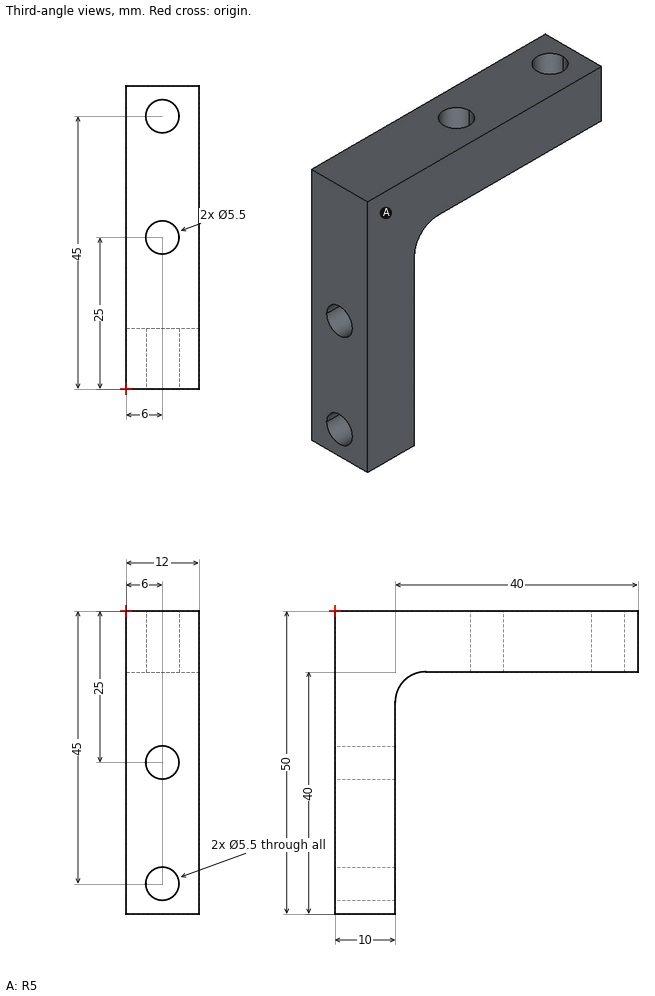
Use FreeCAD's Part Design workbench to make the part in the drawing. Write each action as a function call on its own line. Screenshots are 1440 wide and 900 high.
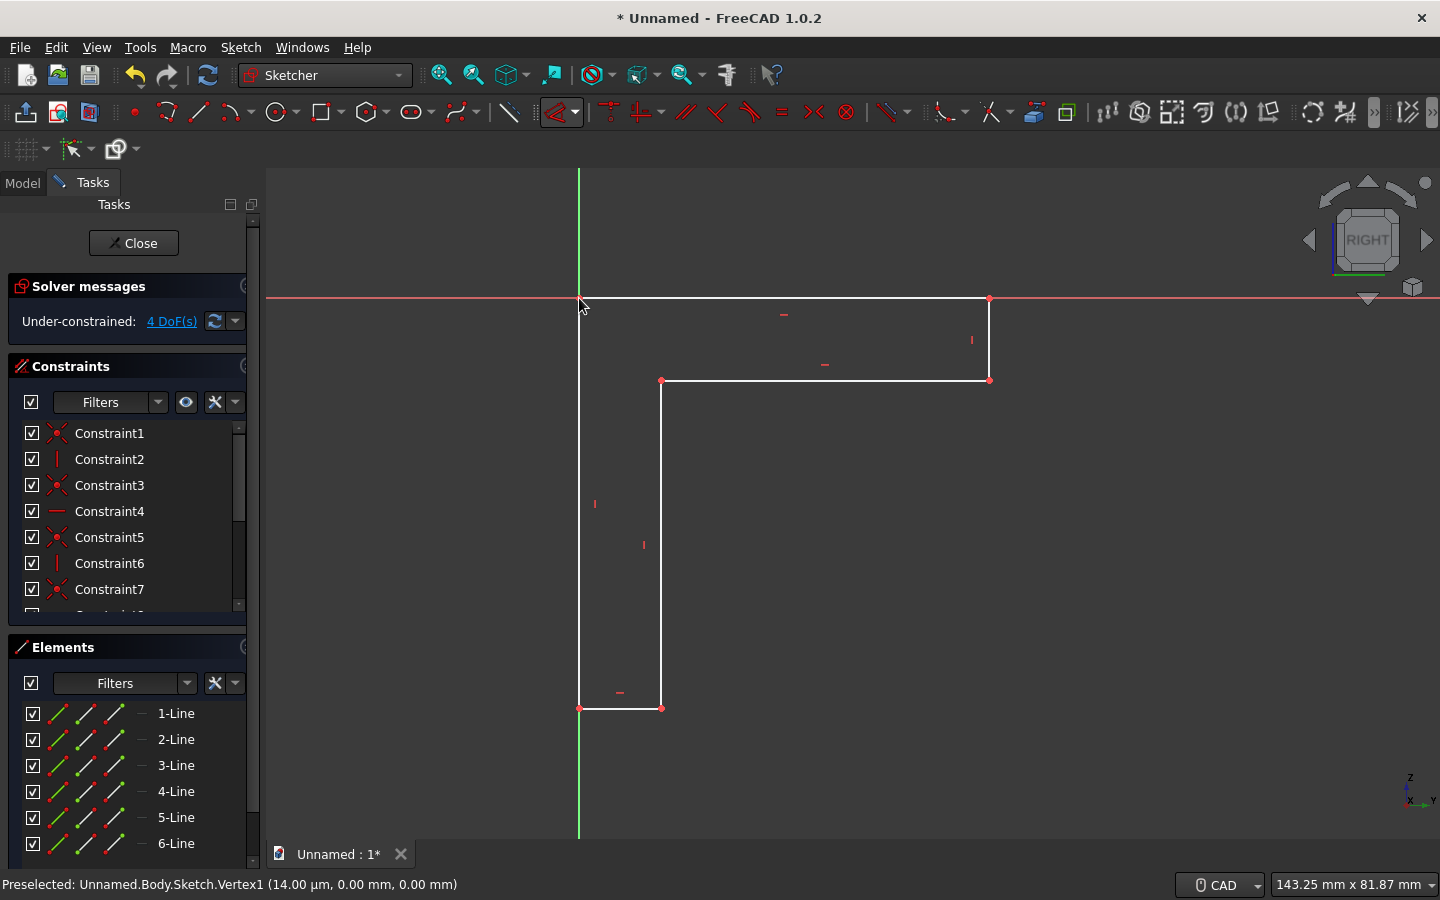
click(556, 112)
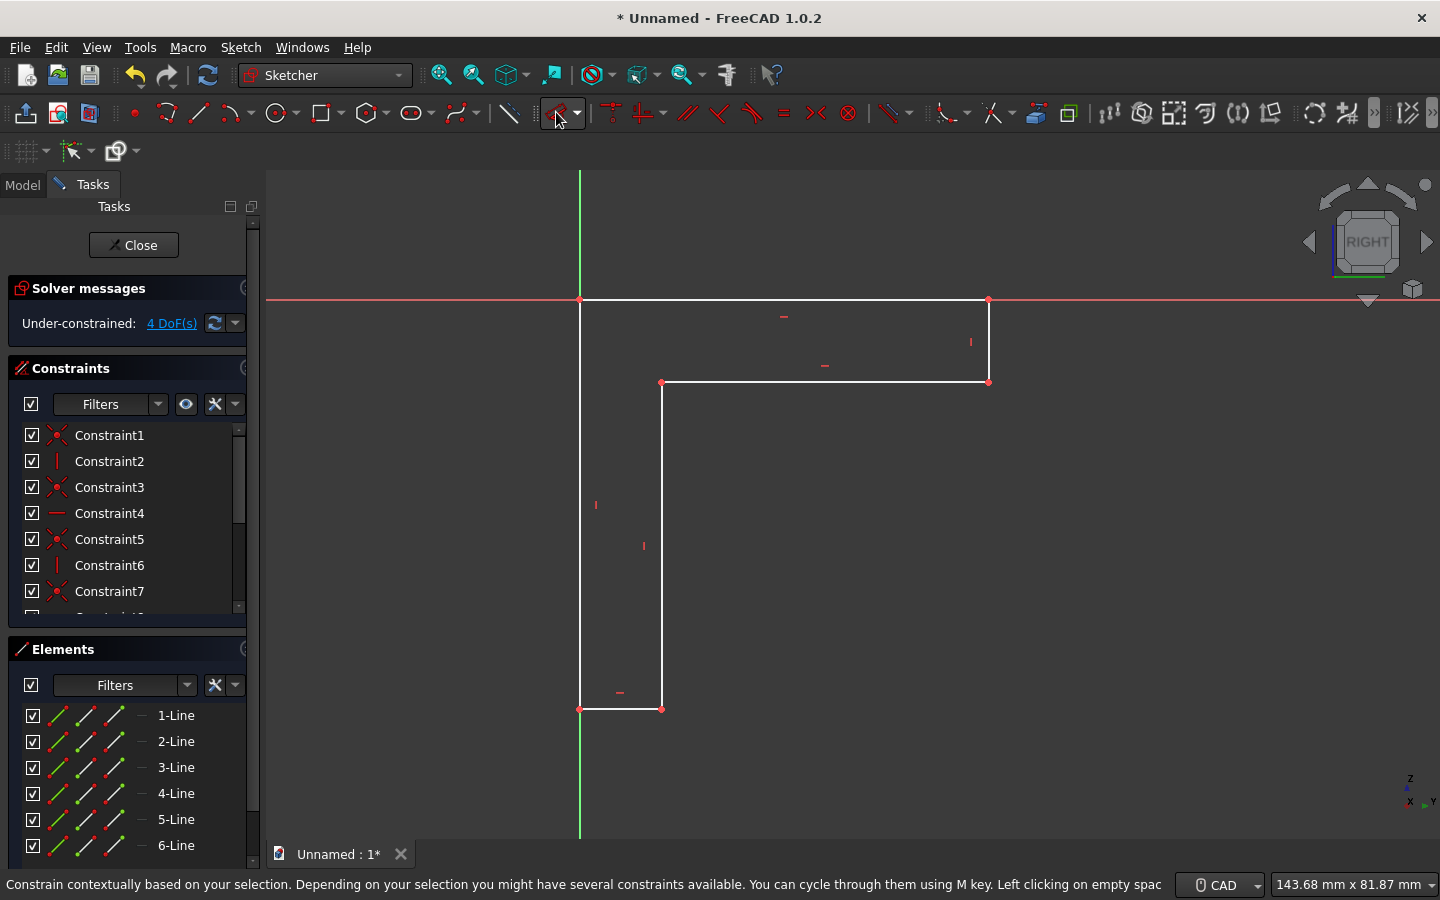
click(580, 423)
click(546, 505)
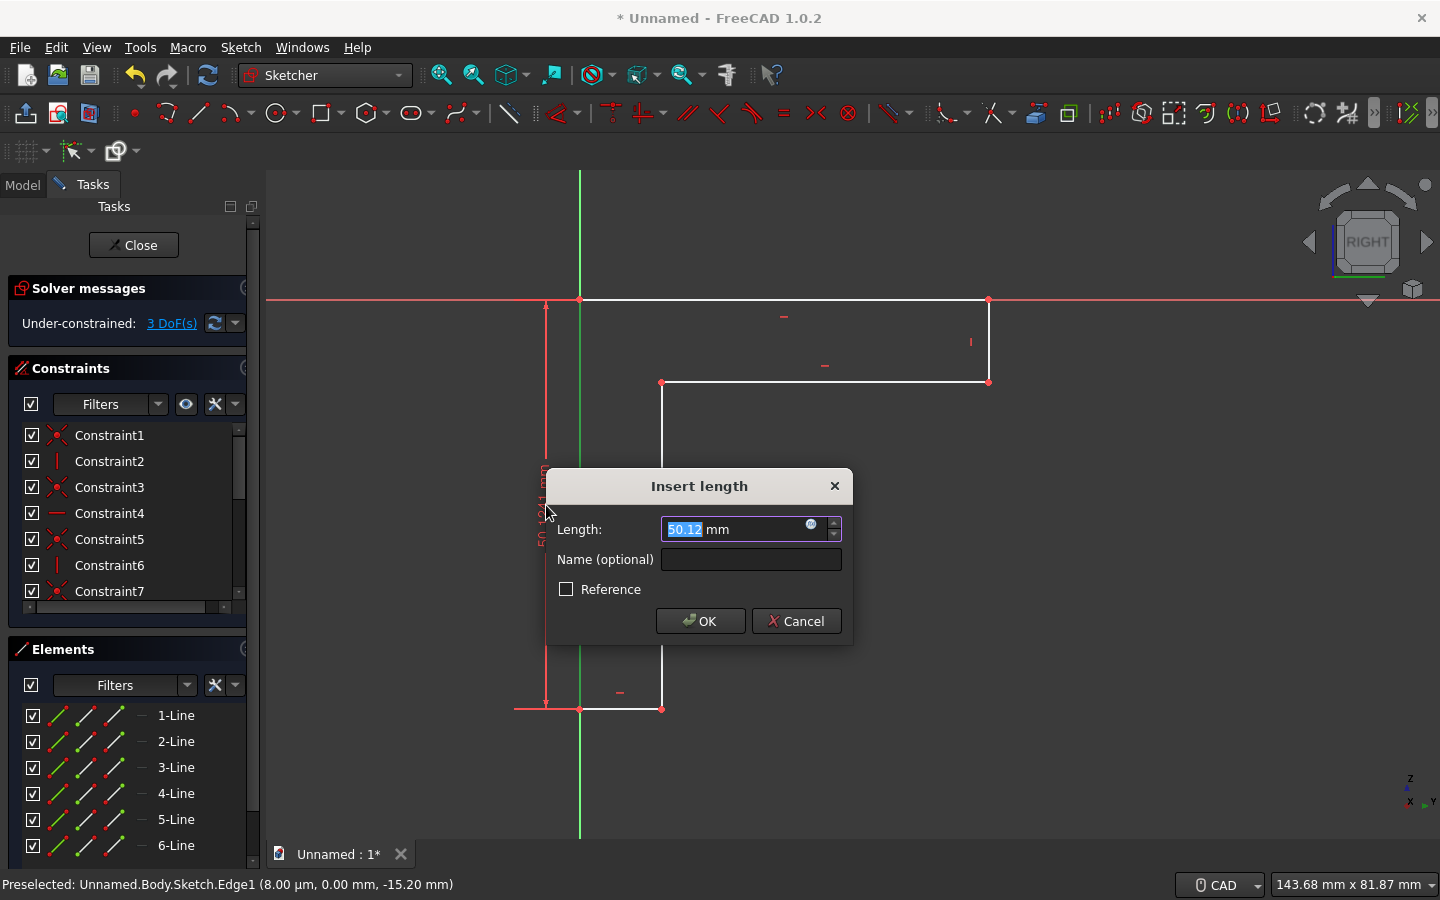
text(50)
key(Return)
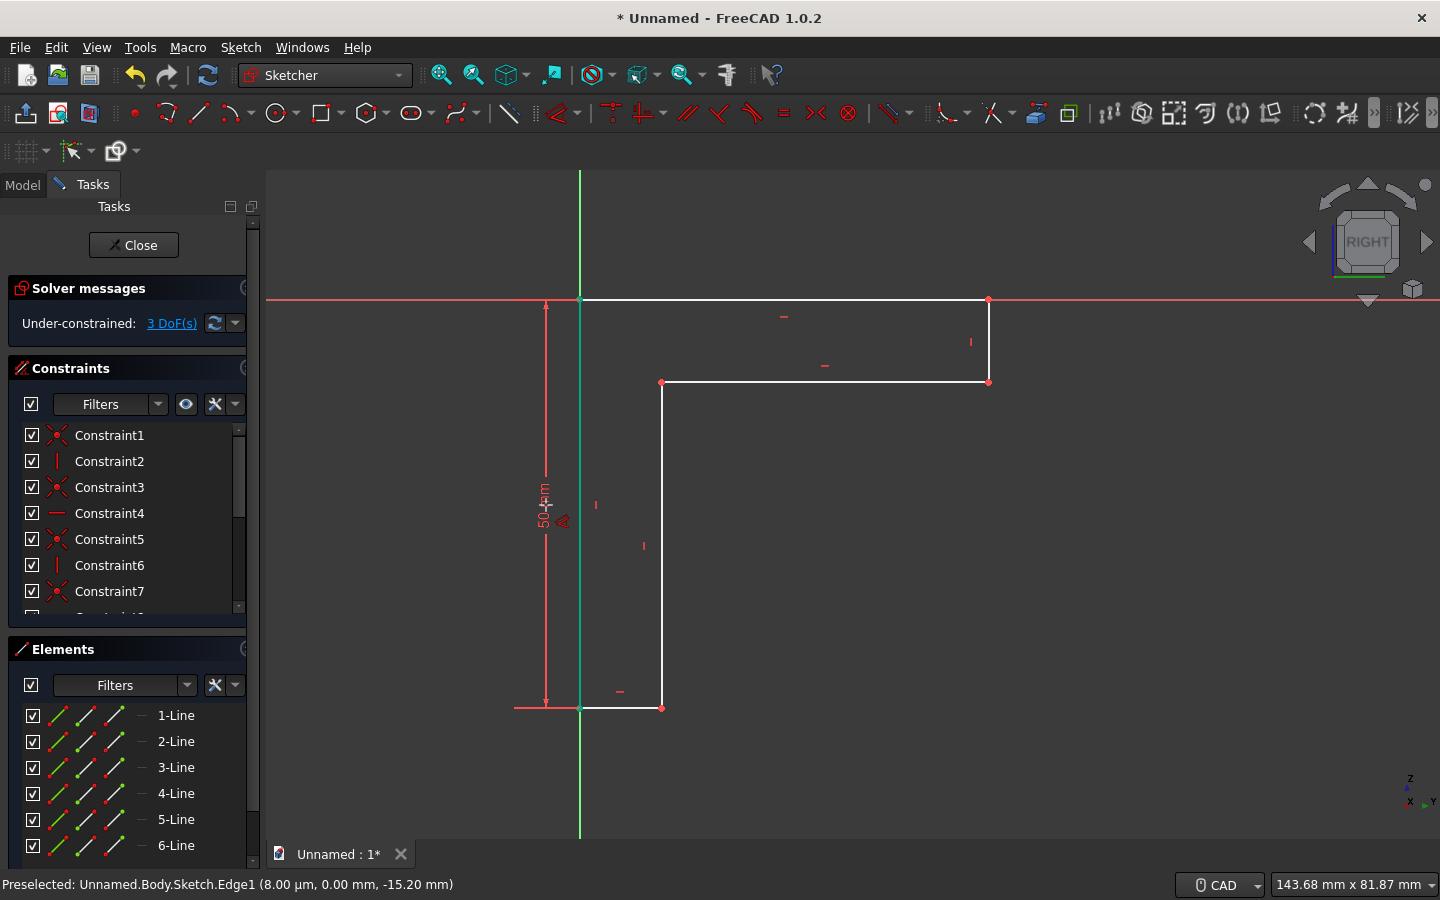
click(604, 708)
click(621, 742)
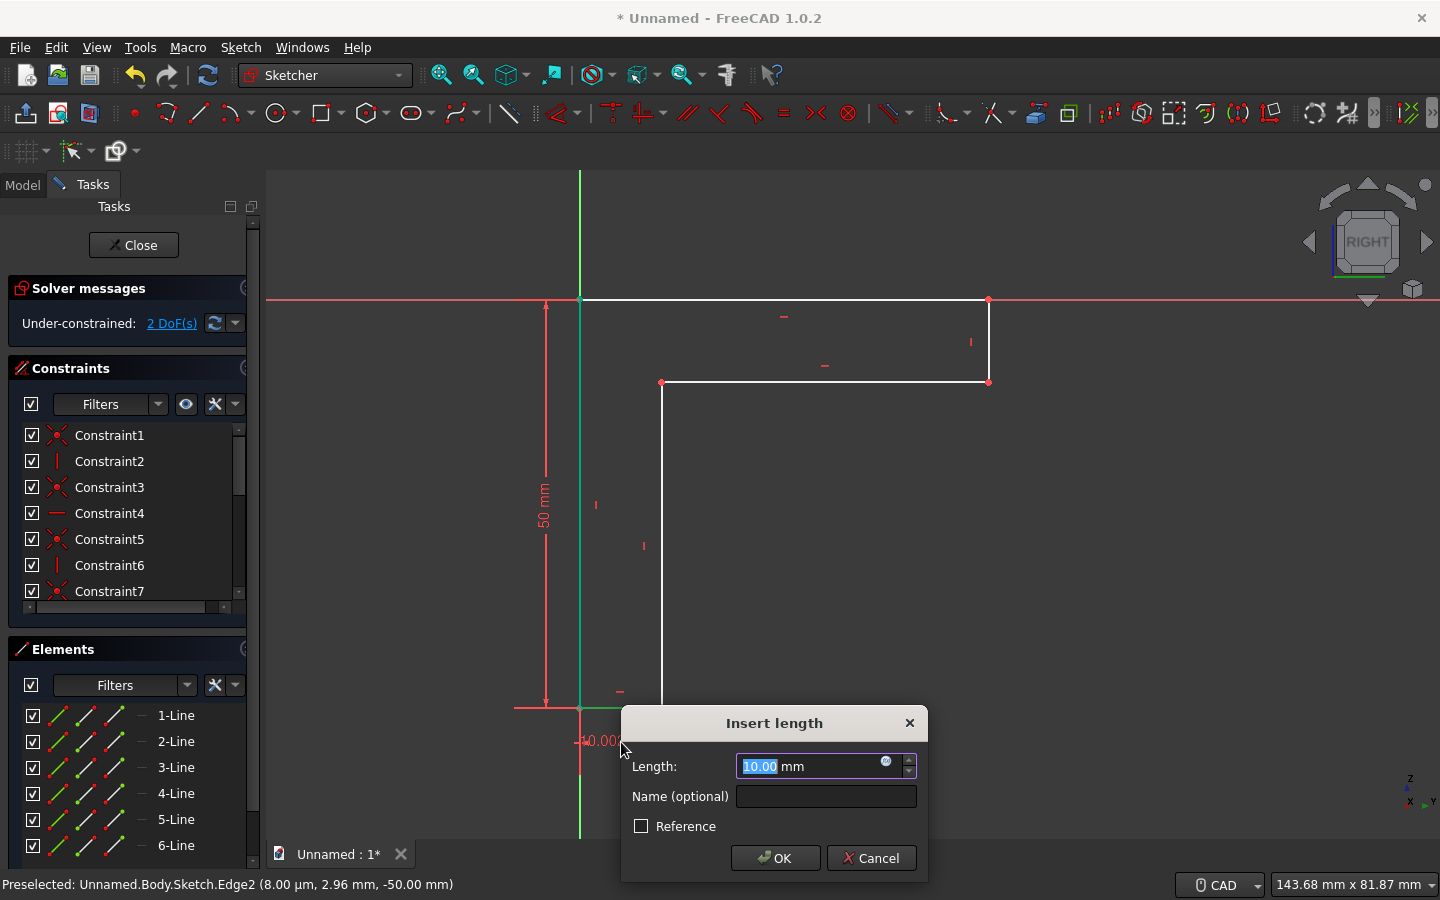
text(10)
key(Return)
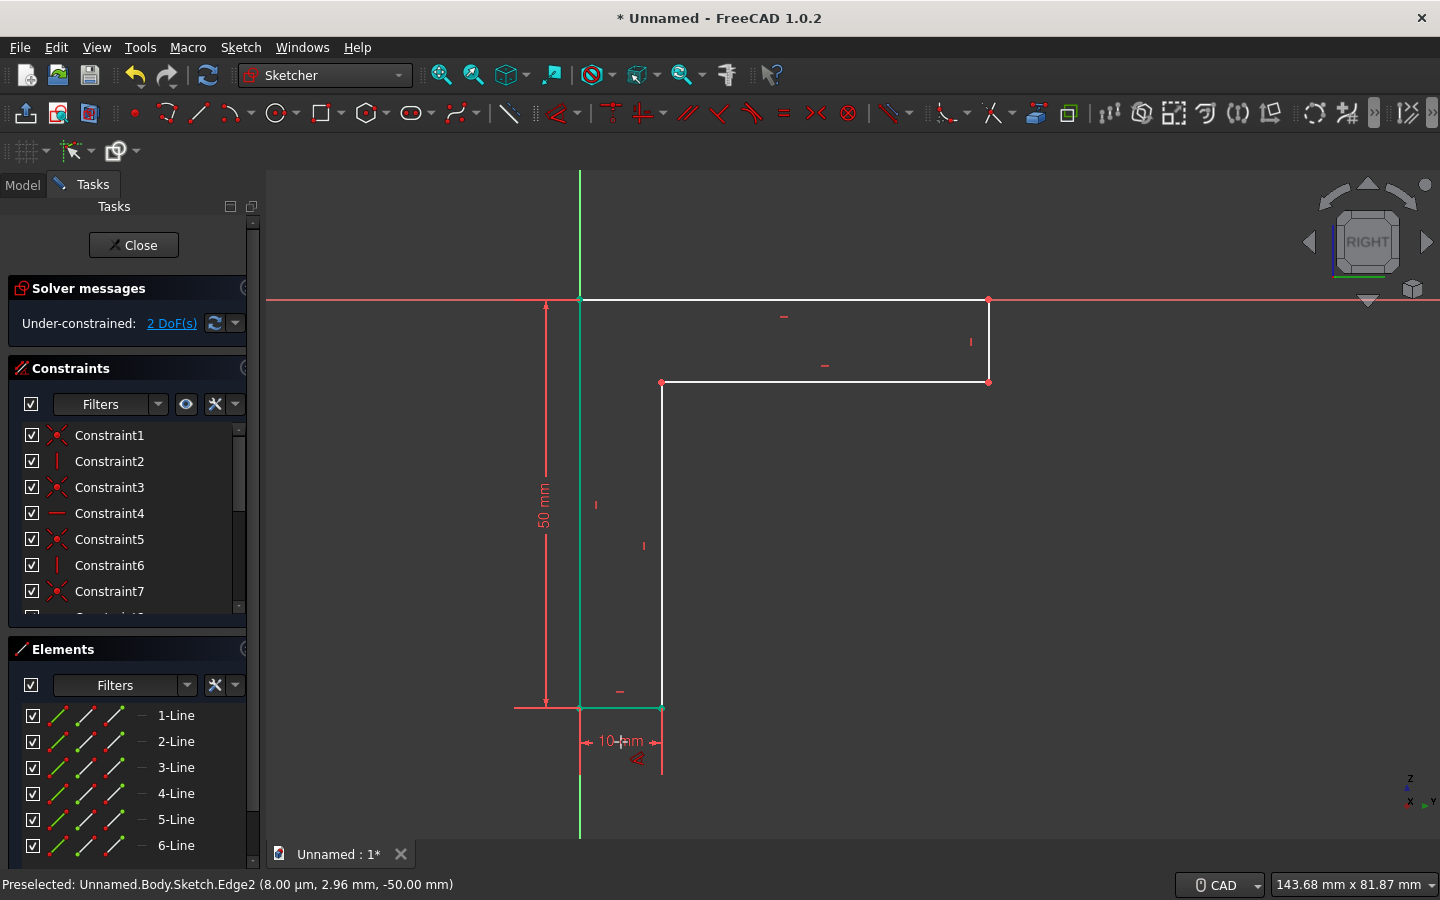
click(662, 611)
click(628, 545)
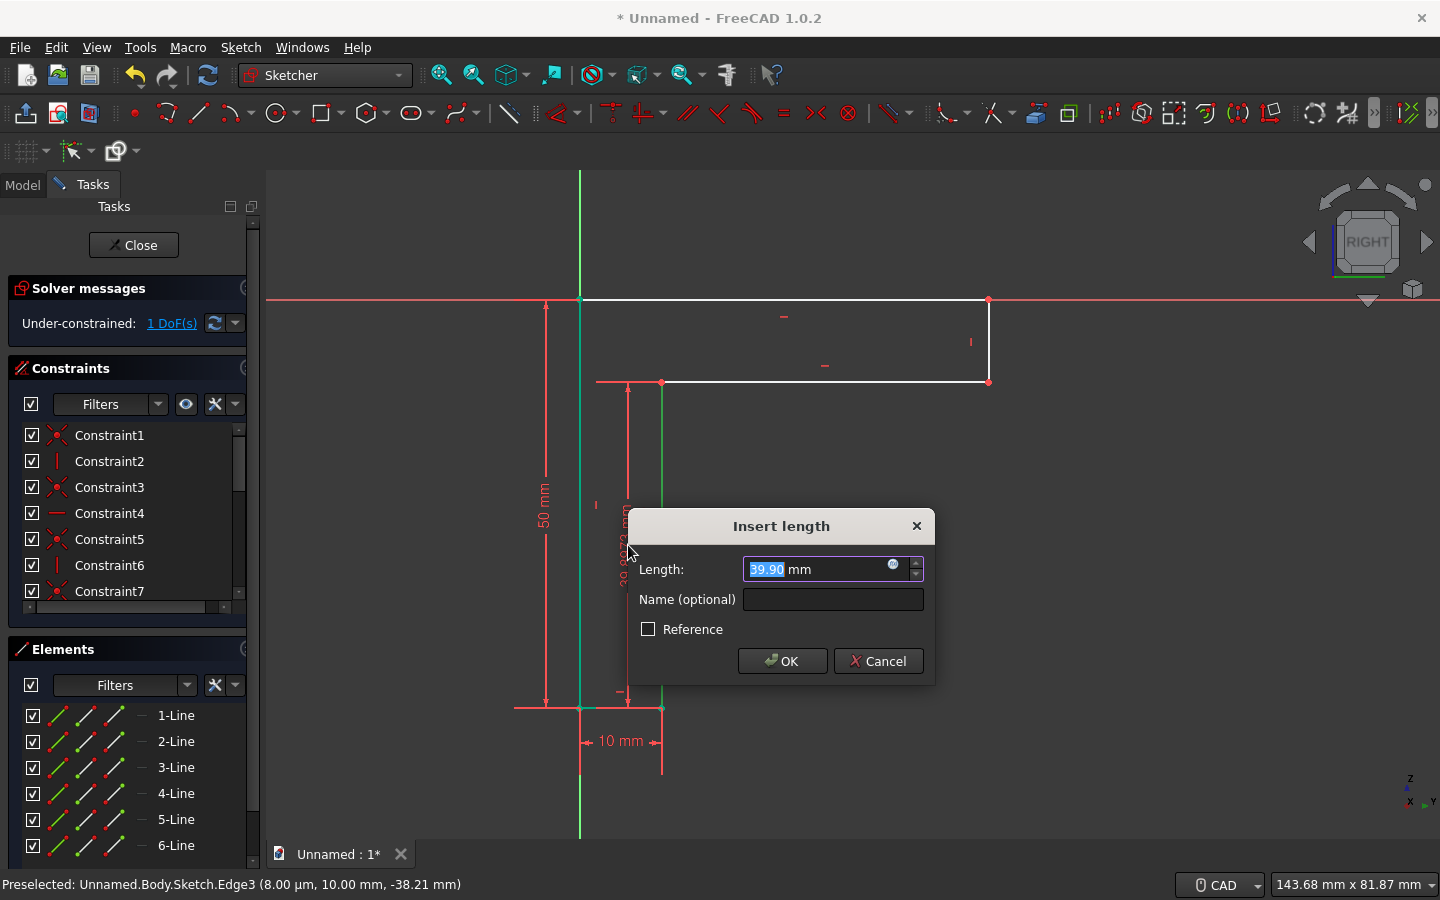
text(40)
key(Return)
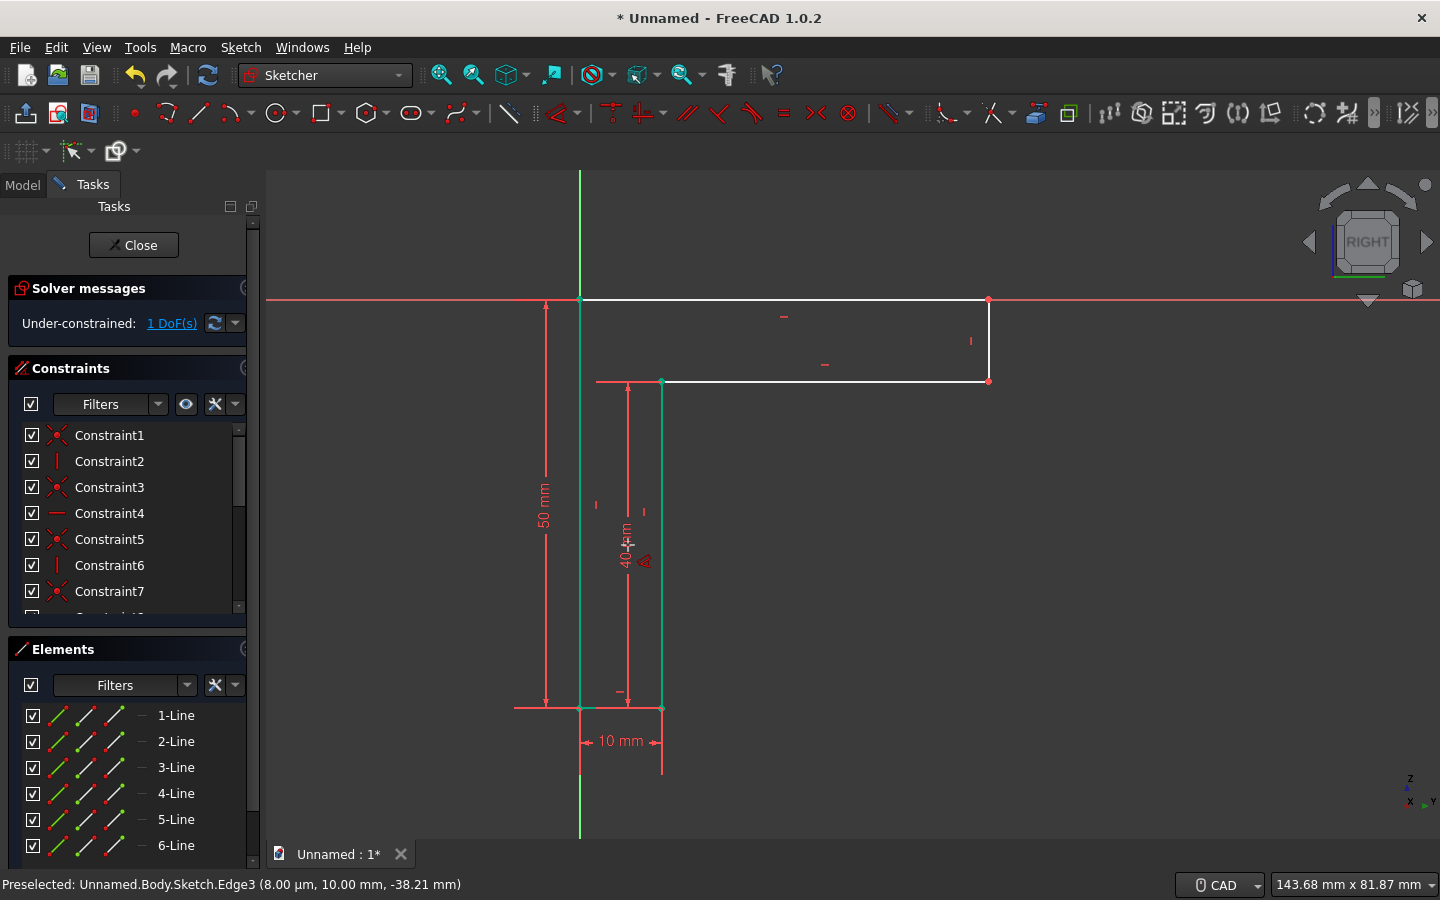
click(760, 382)
click(825, 348)